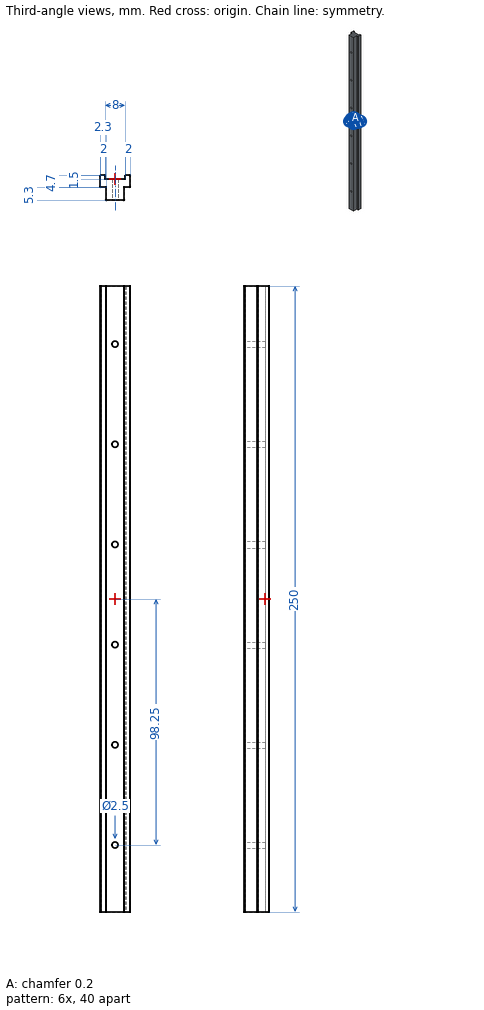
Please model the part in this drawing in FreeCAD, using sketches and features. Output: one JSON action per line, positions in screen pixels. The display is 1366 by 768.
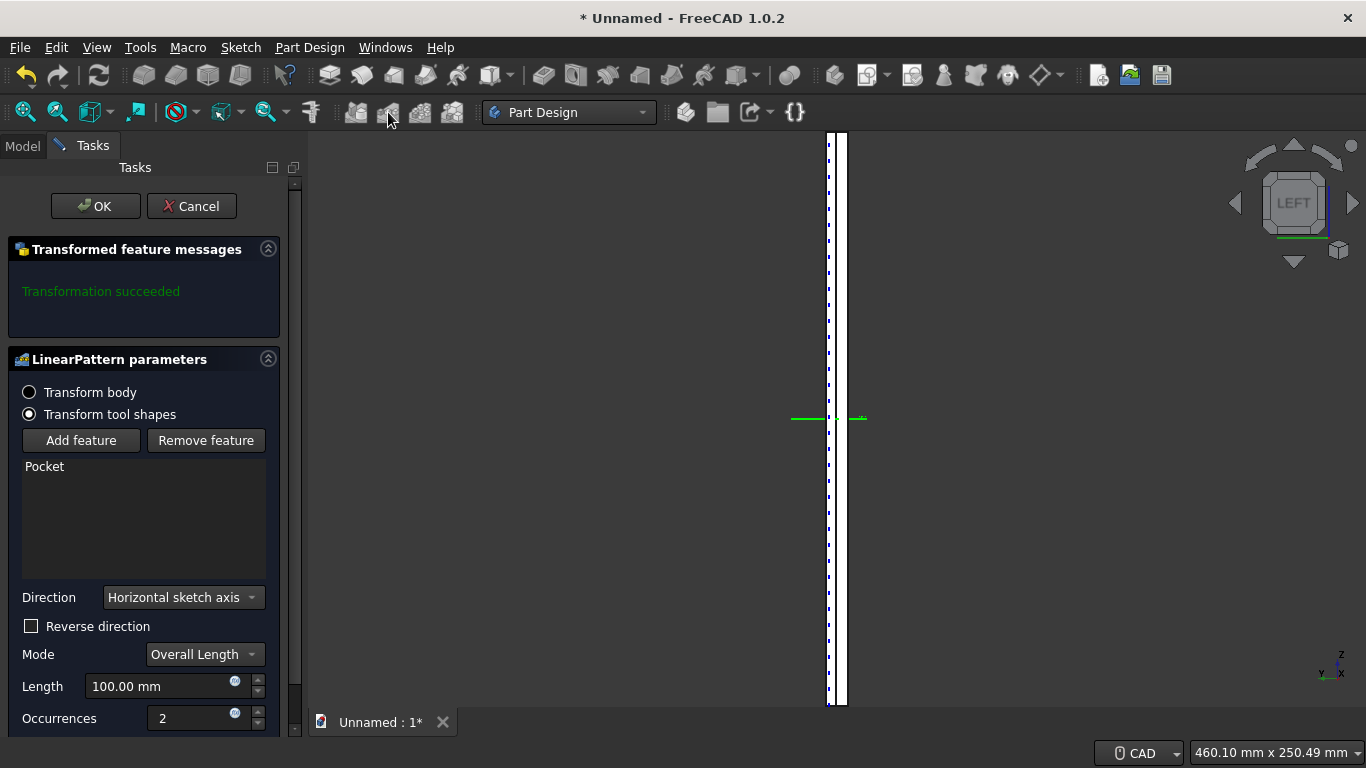
{"action": "left_click", "coordinate": [184, 598]}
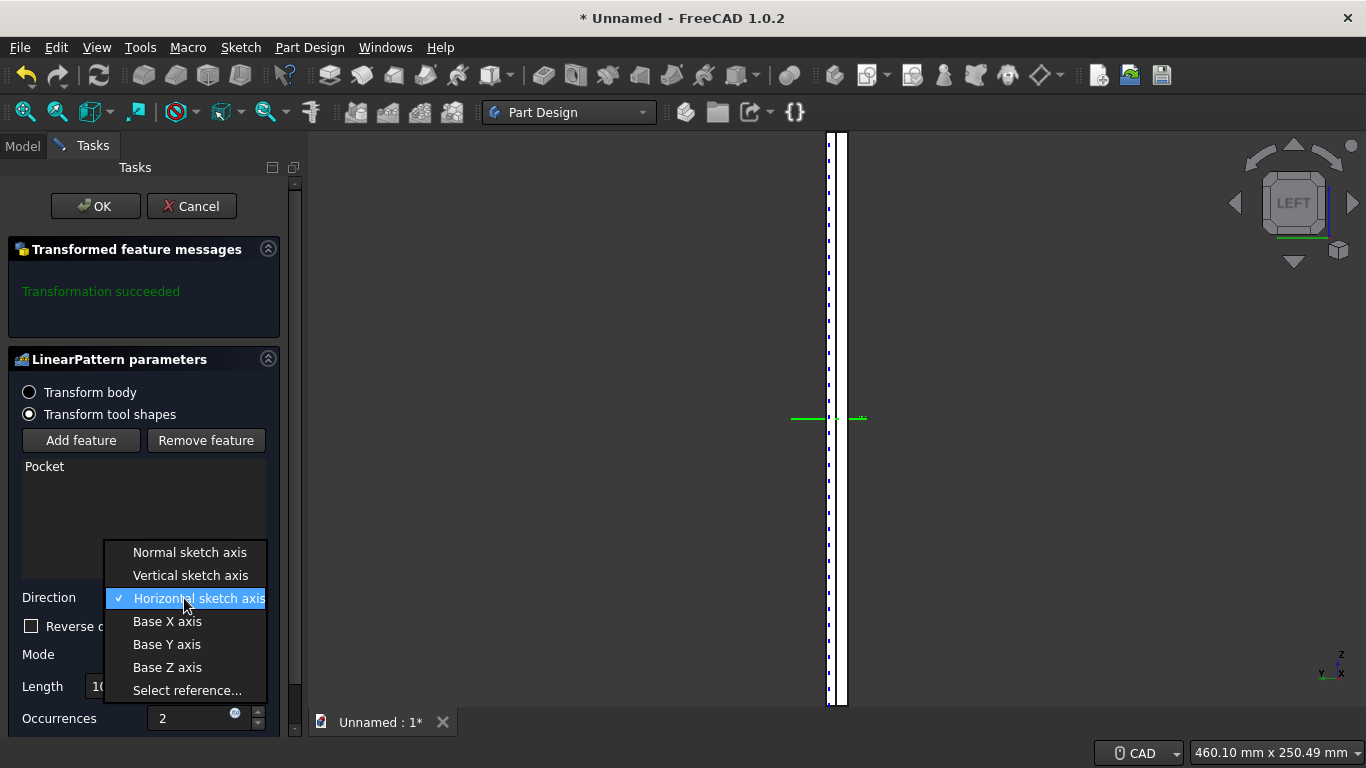
{"action": "left_click", "coordinate": [184, 668]}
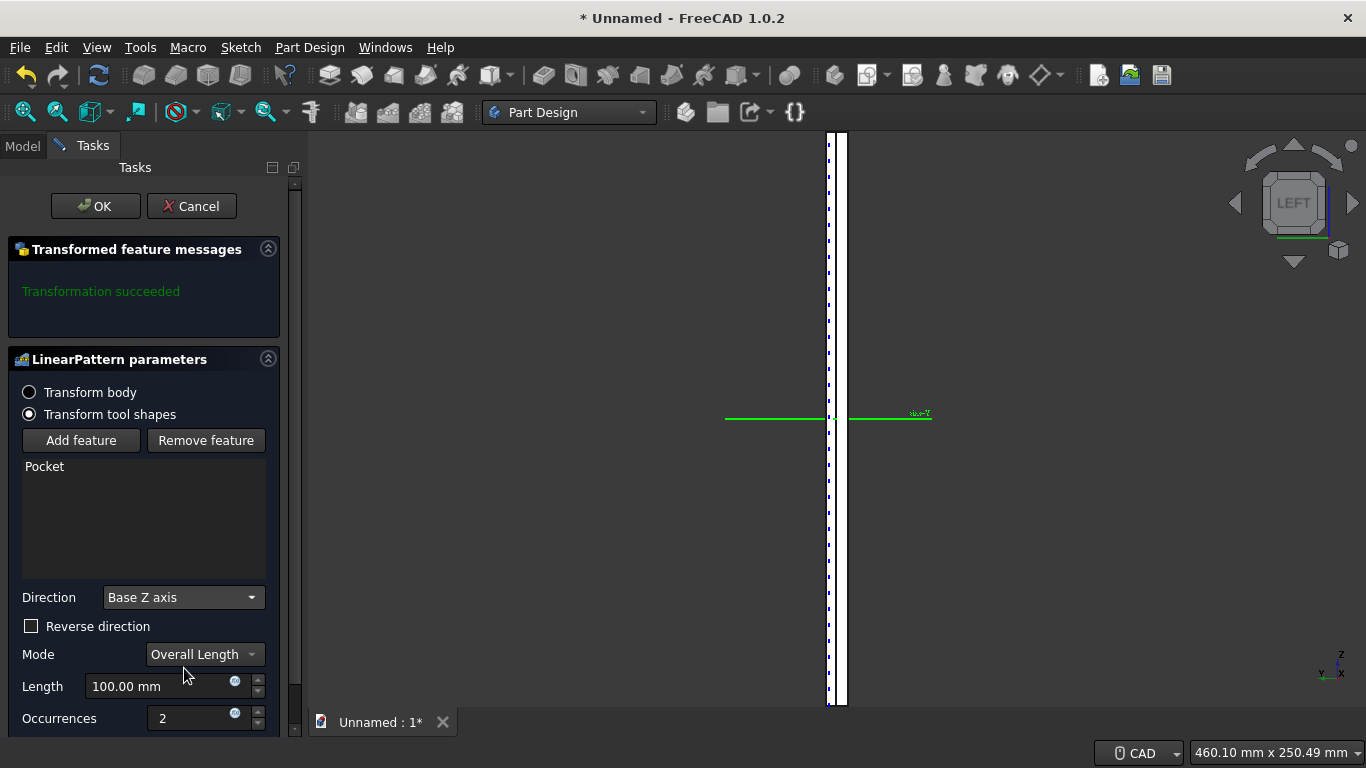
{"action": "left_click", "coordinate": [206, 654]}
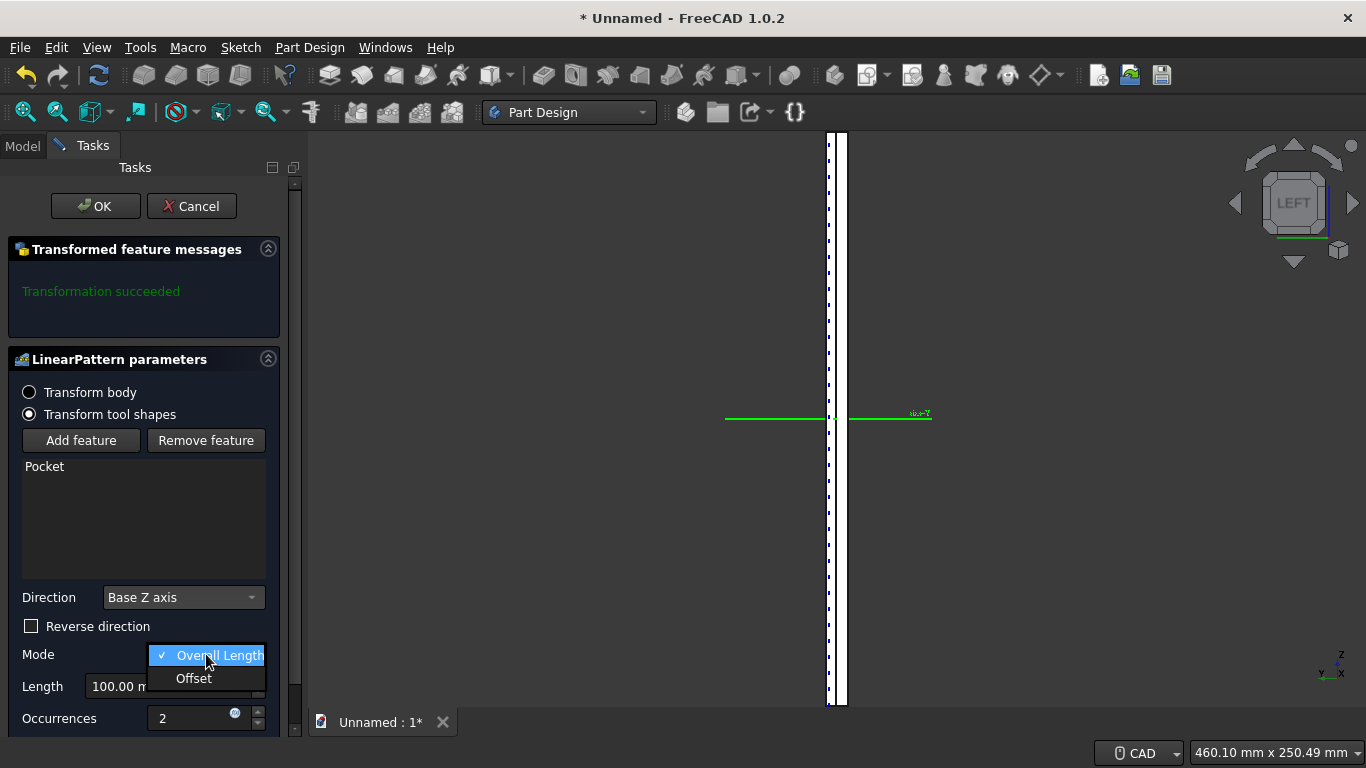
{"action": "left_click", "coordinate": [206, 678]}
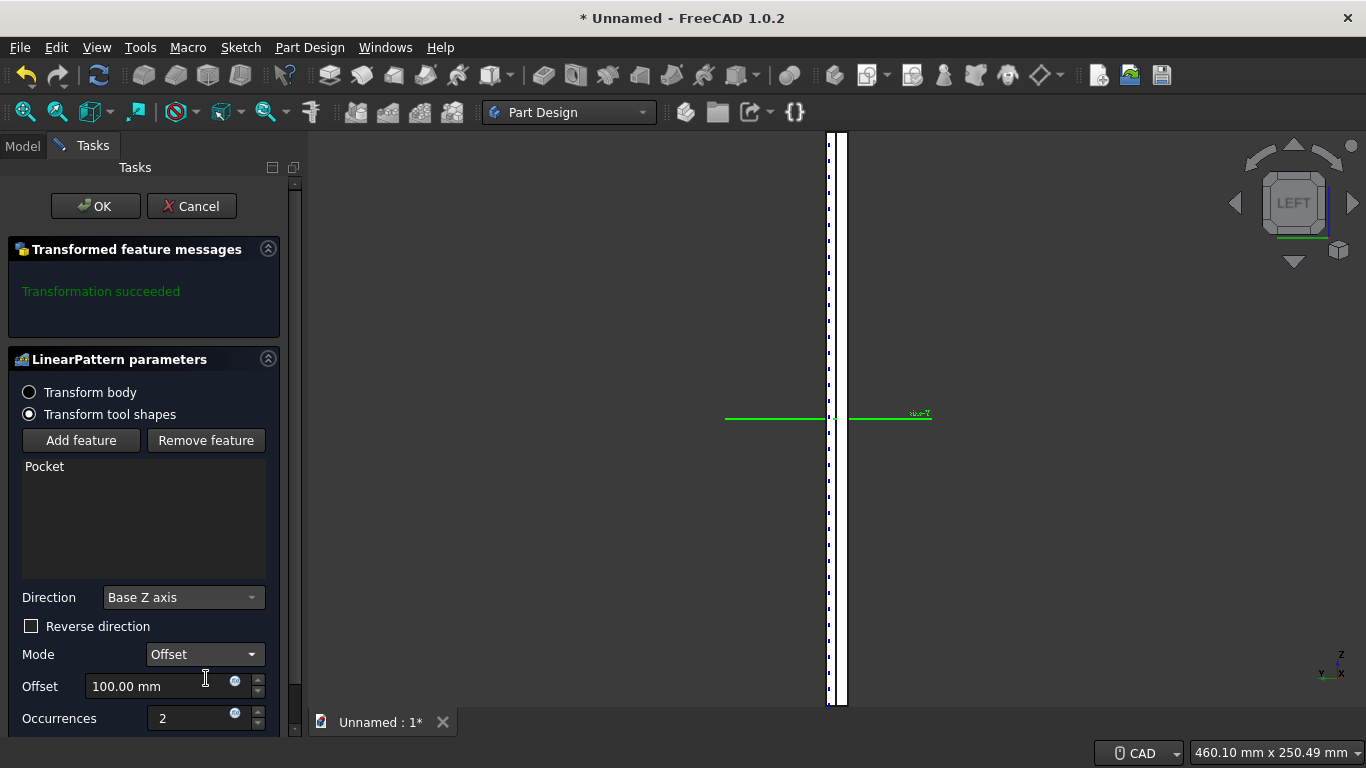
{"action": "triple_click", "coordinate": [168, 686]}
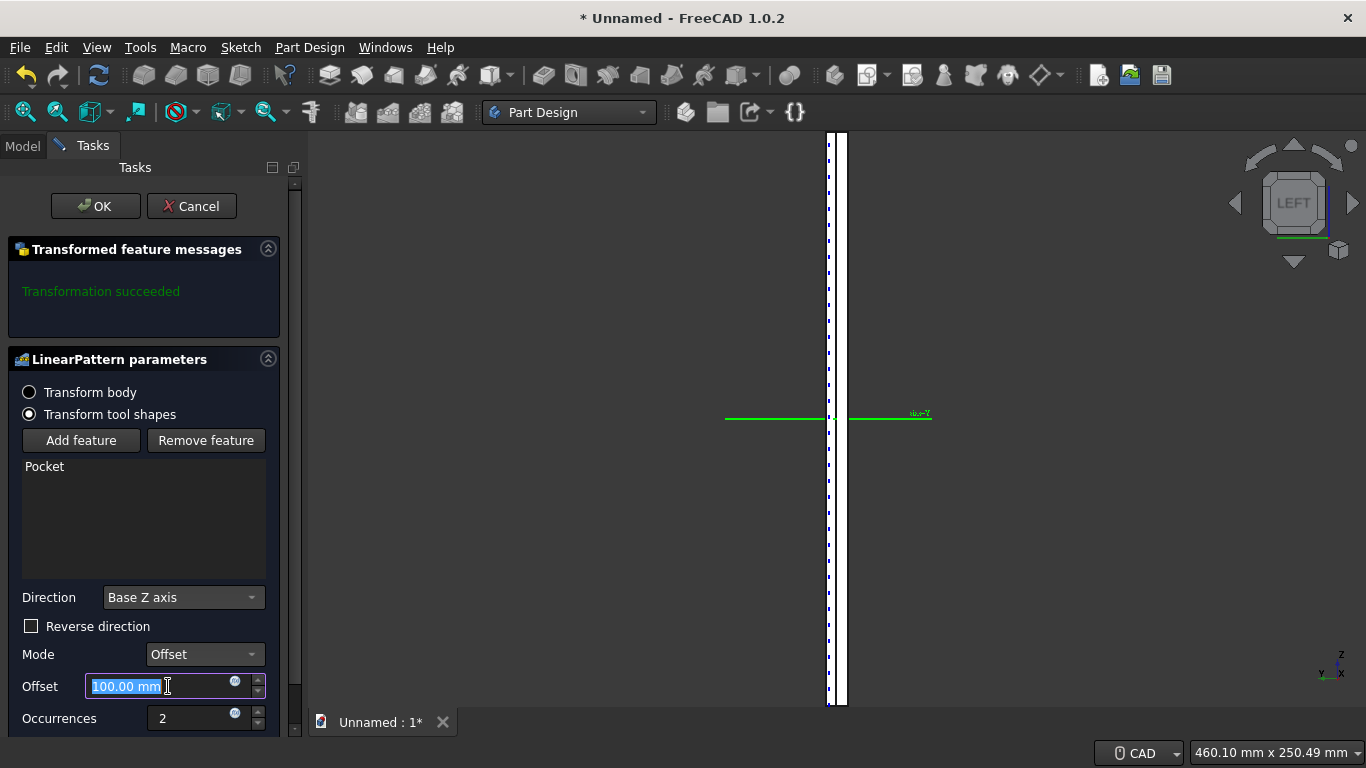
{"action": "type", "text": "40"}
{"action": "key", "text": "Tab"}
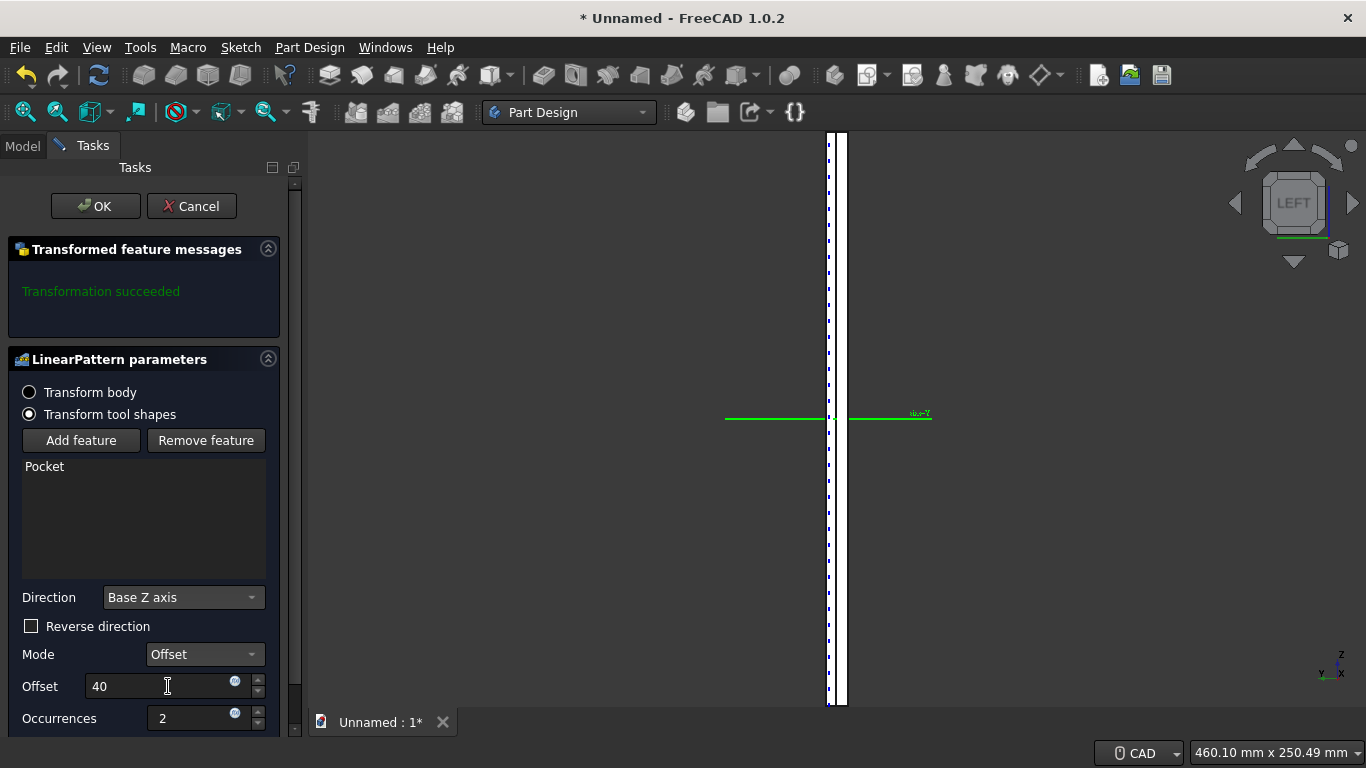
{"action": "triple_click", "coordinate": [198, 718]}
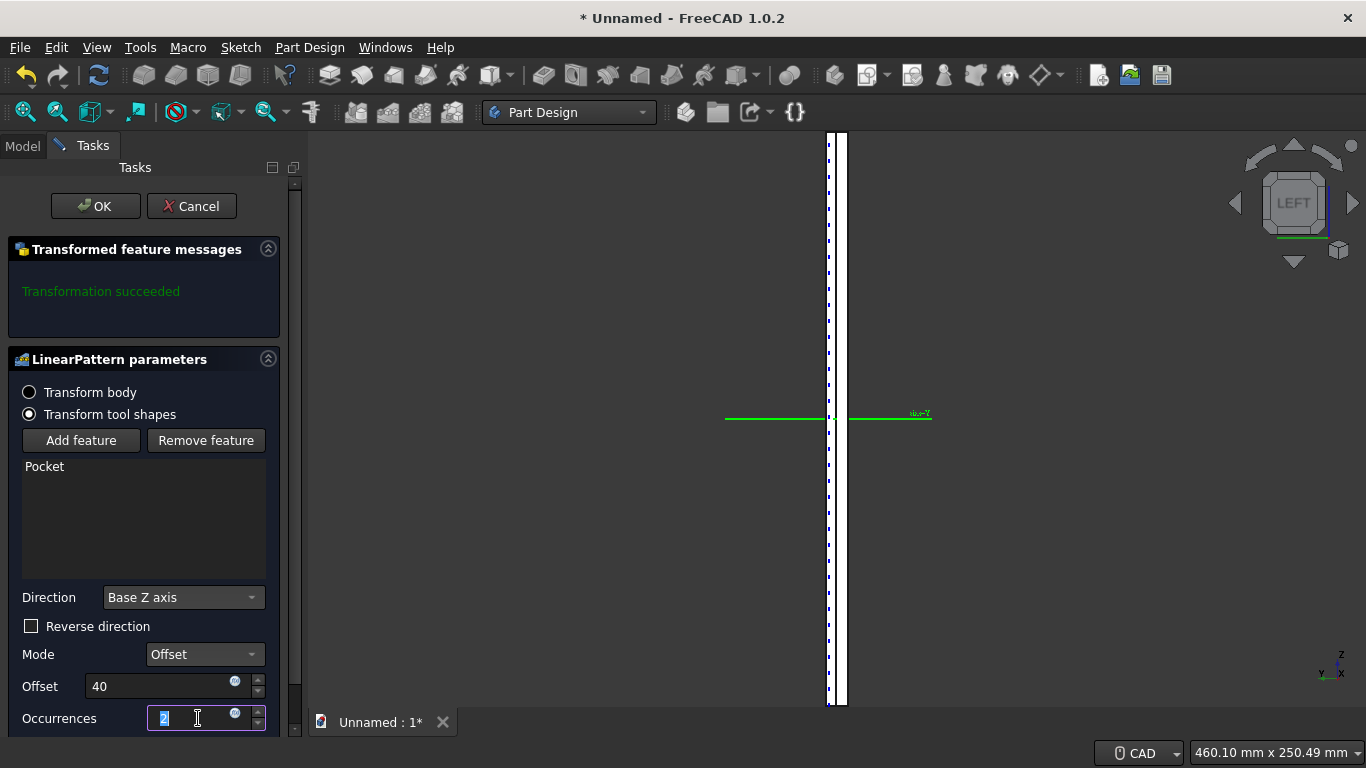
{"action": "type", "text": "6"}
{"action": "key", "text": "Tab"}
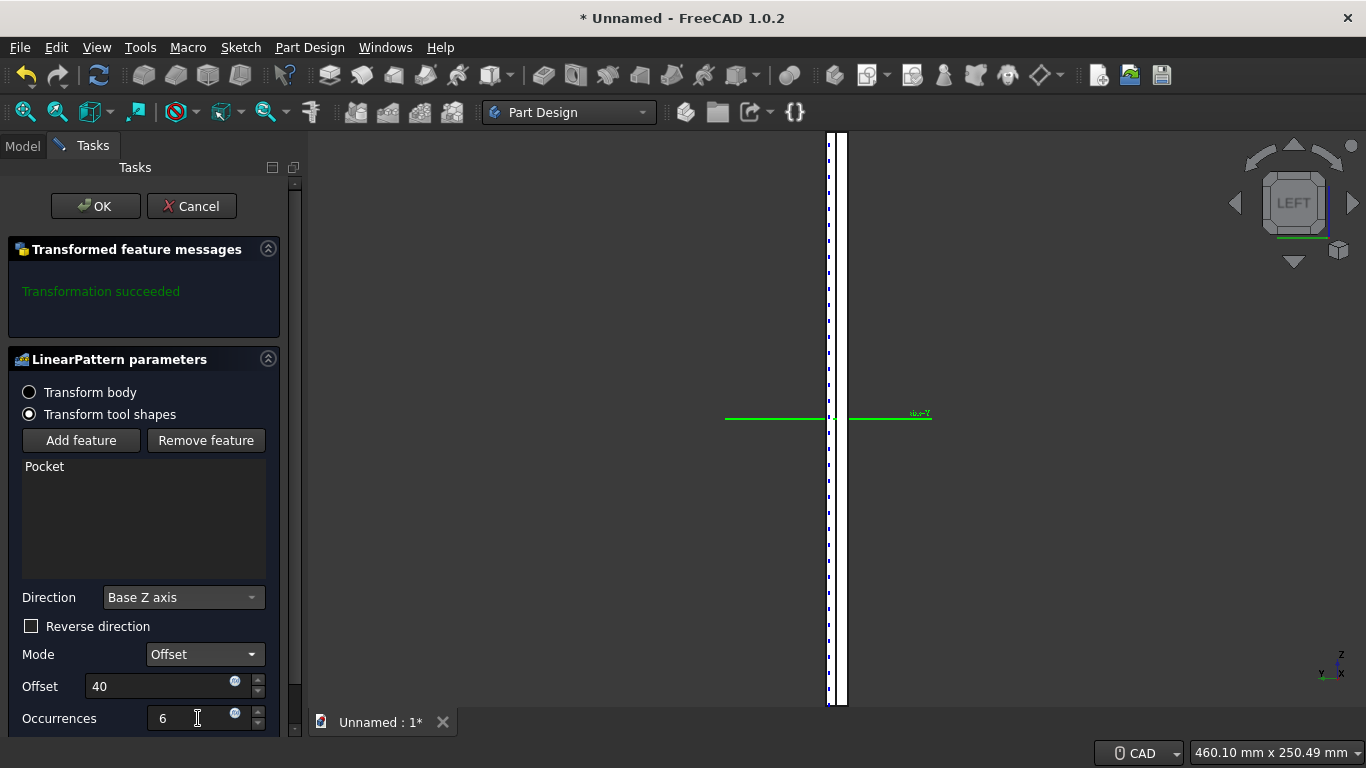
{"action": "left_click", "coordinate": [96, 206]}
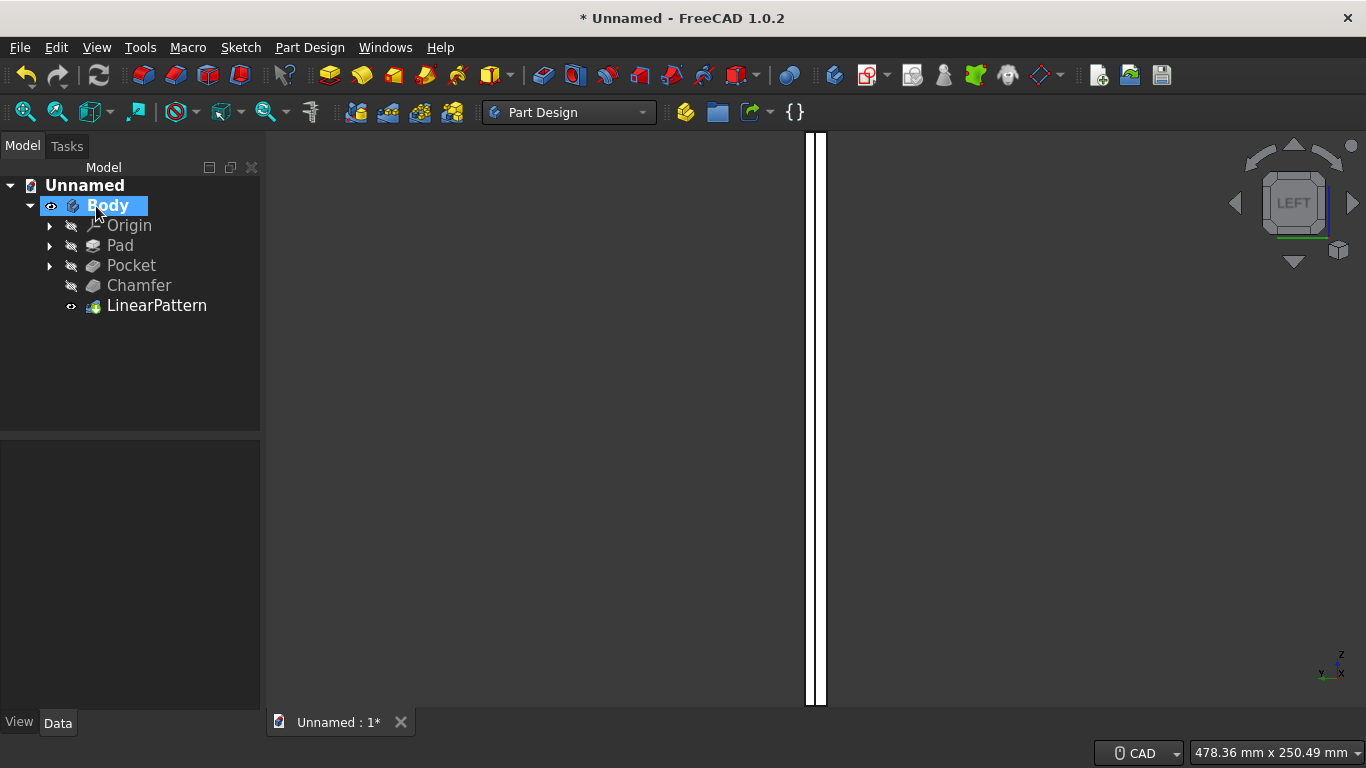
{"action": "key", "text": "0"}